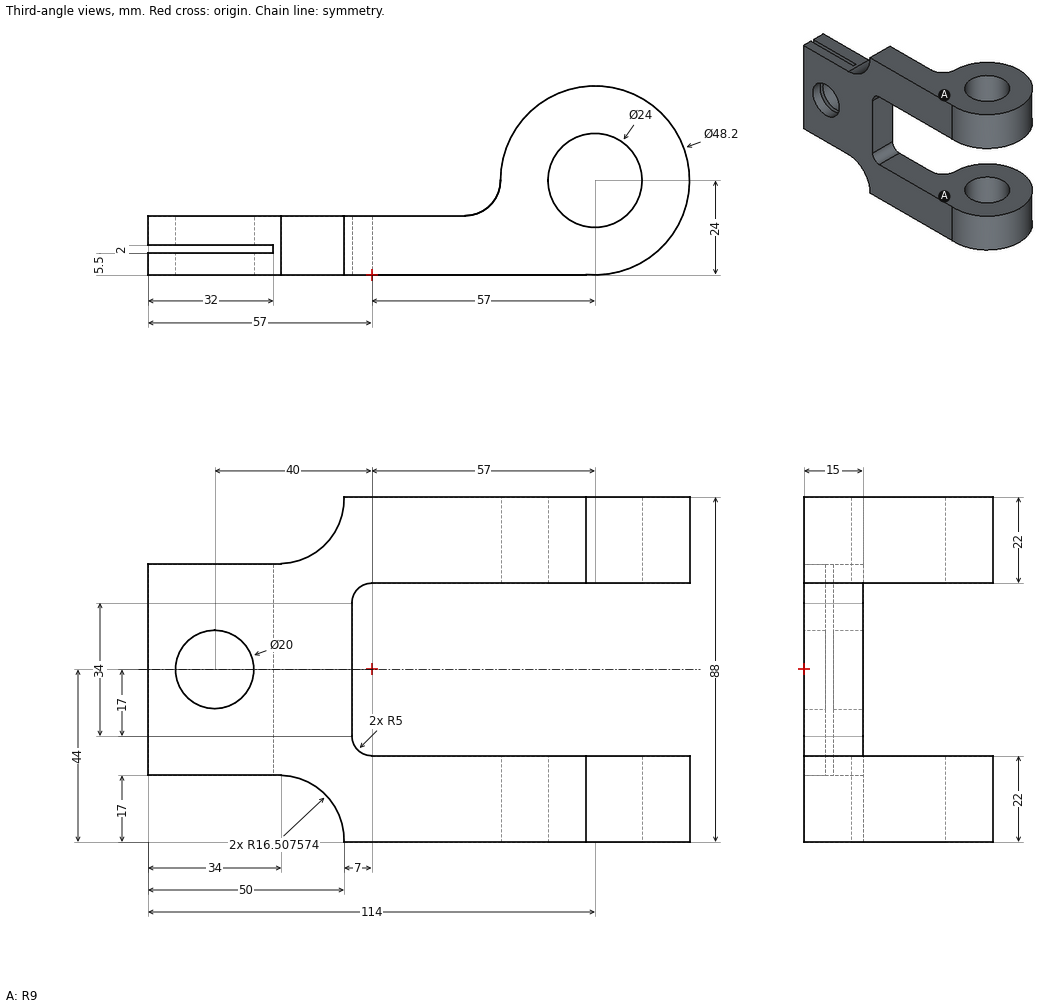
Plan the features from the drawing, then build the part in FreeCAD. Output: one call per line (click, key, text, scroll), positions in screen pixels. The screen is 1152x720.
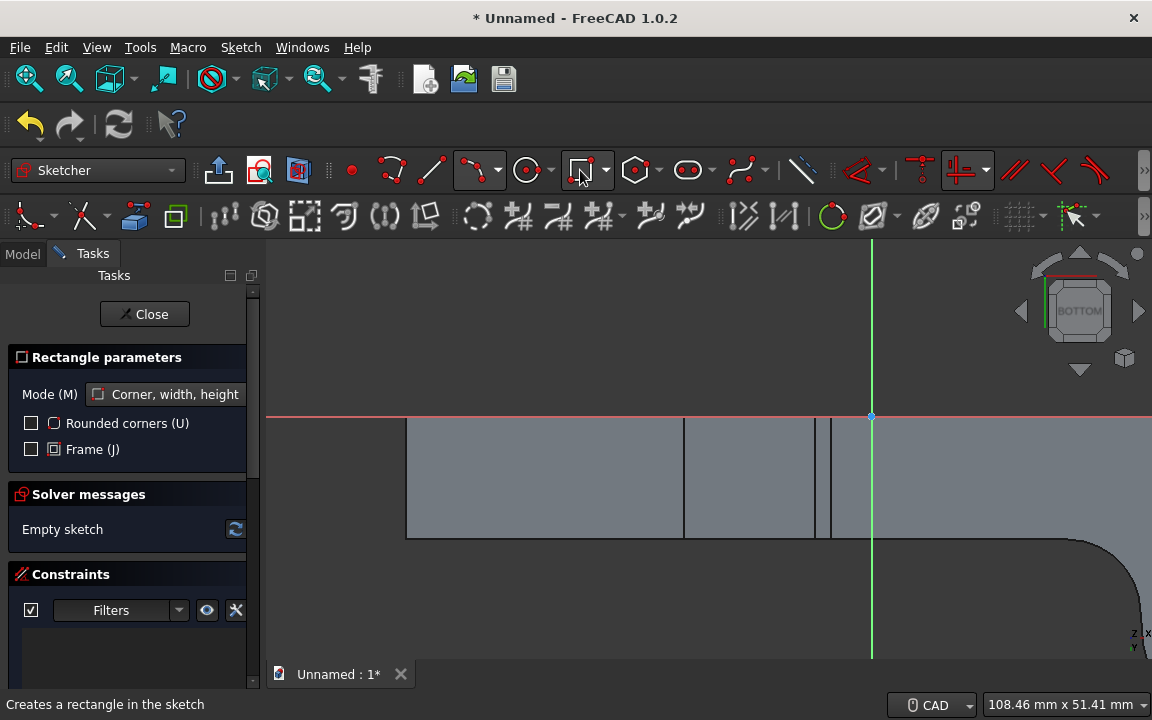
click(406, 462)
move(668, 478)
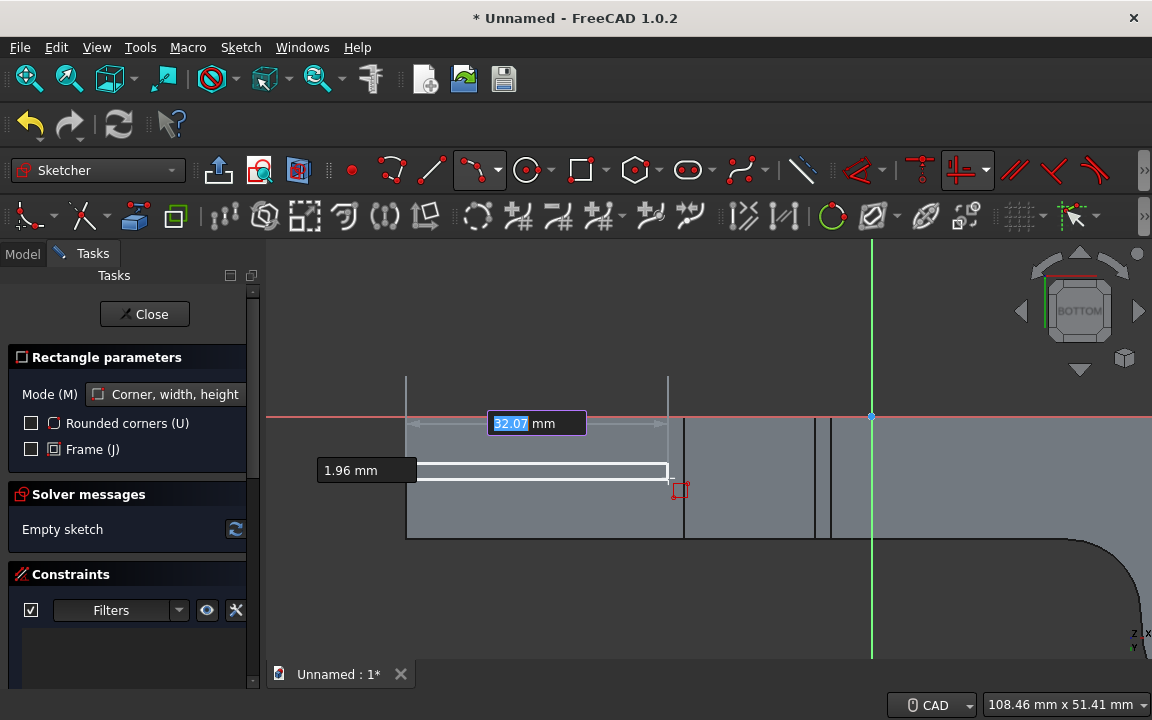
text(32)
key(Tab)
text(2)
key(Return)
key(Escape)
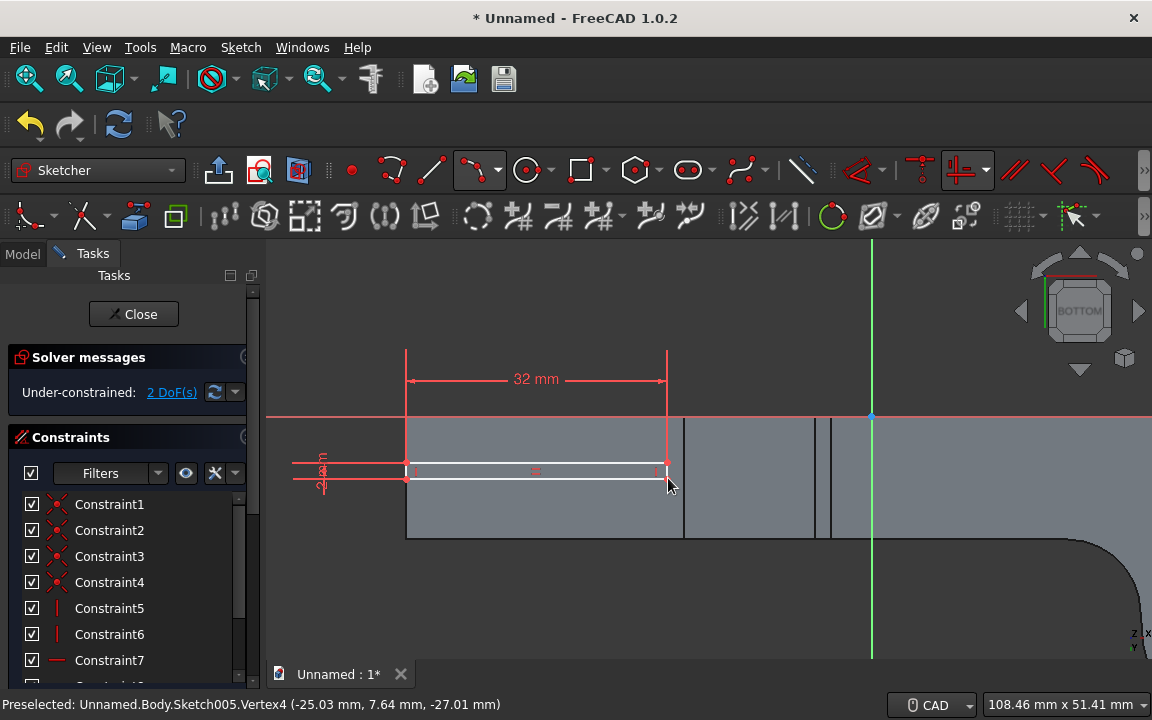
key(d)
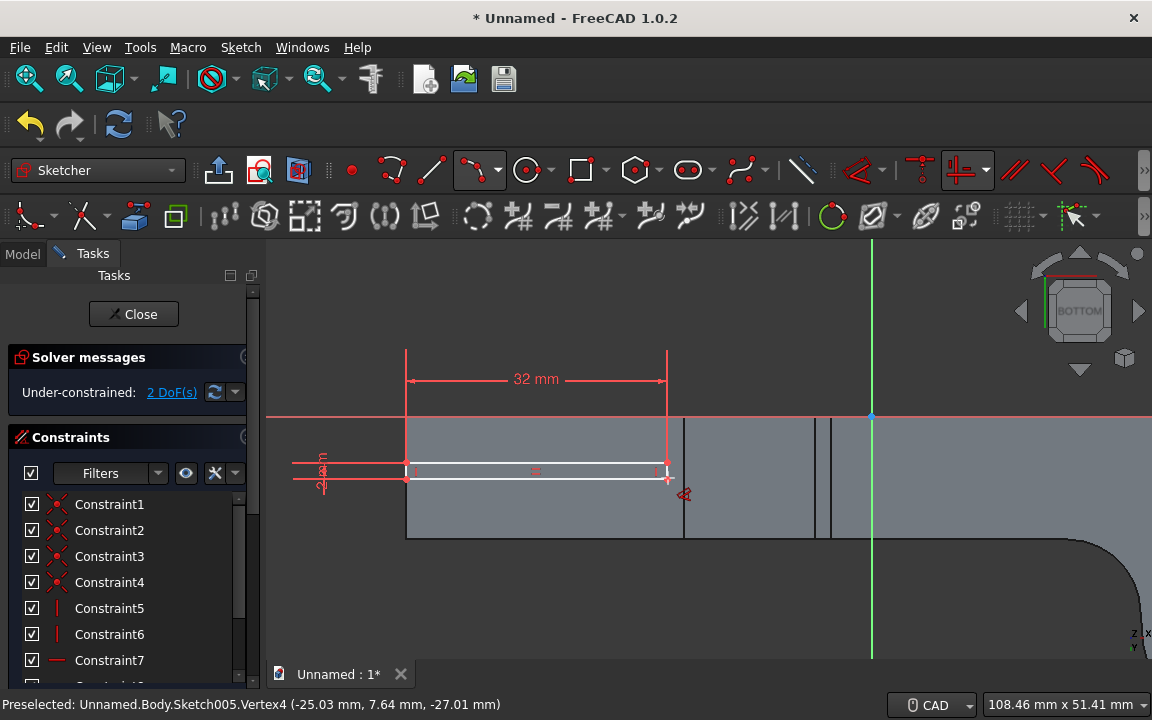
click(406, 463)
click(639, 383)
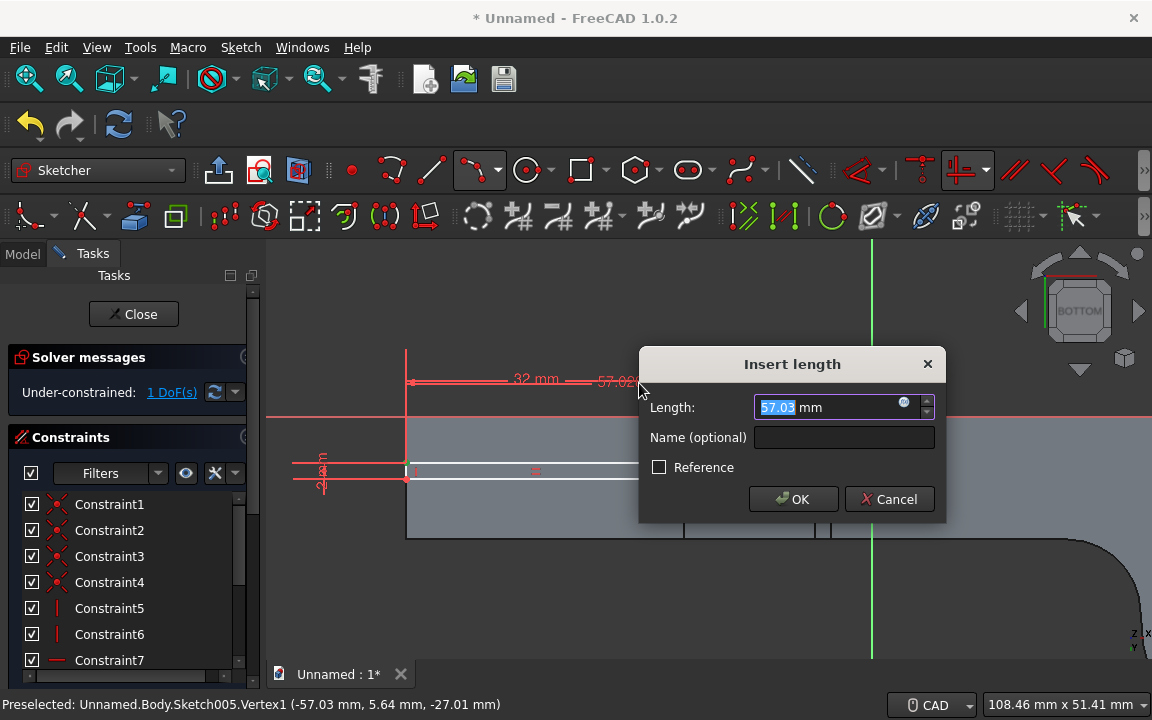
text(57)
key(Return)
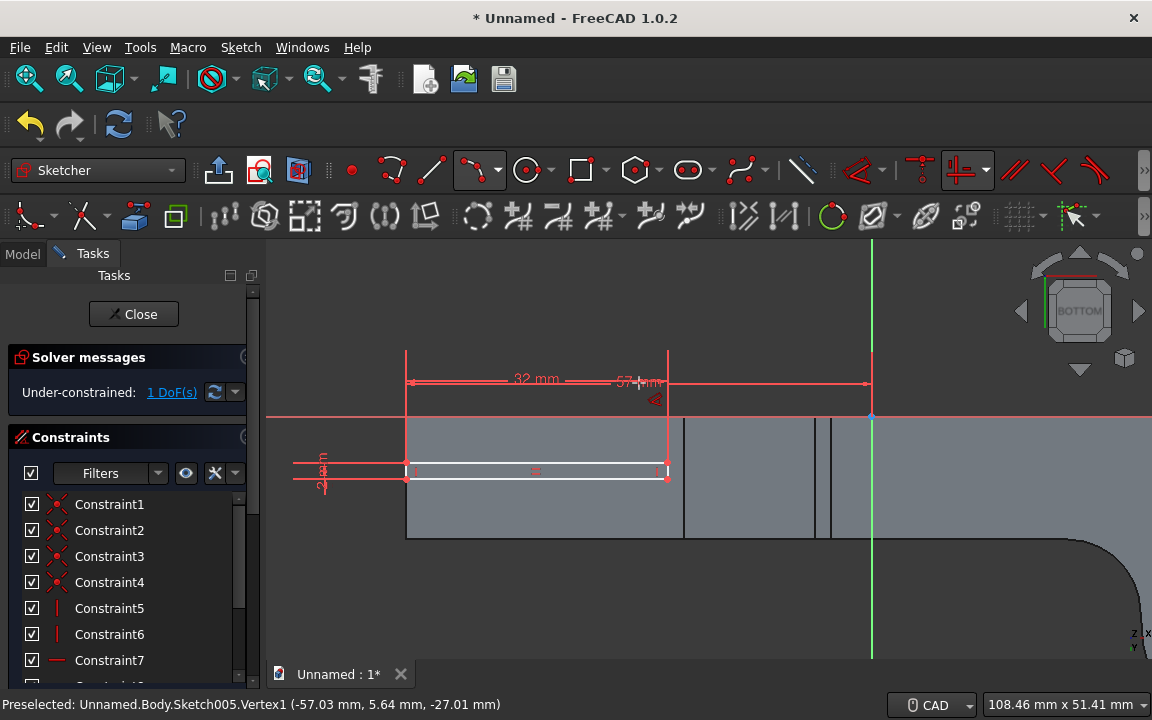
click(406, 463)
click(906, 440)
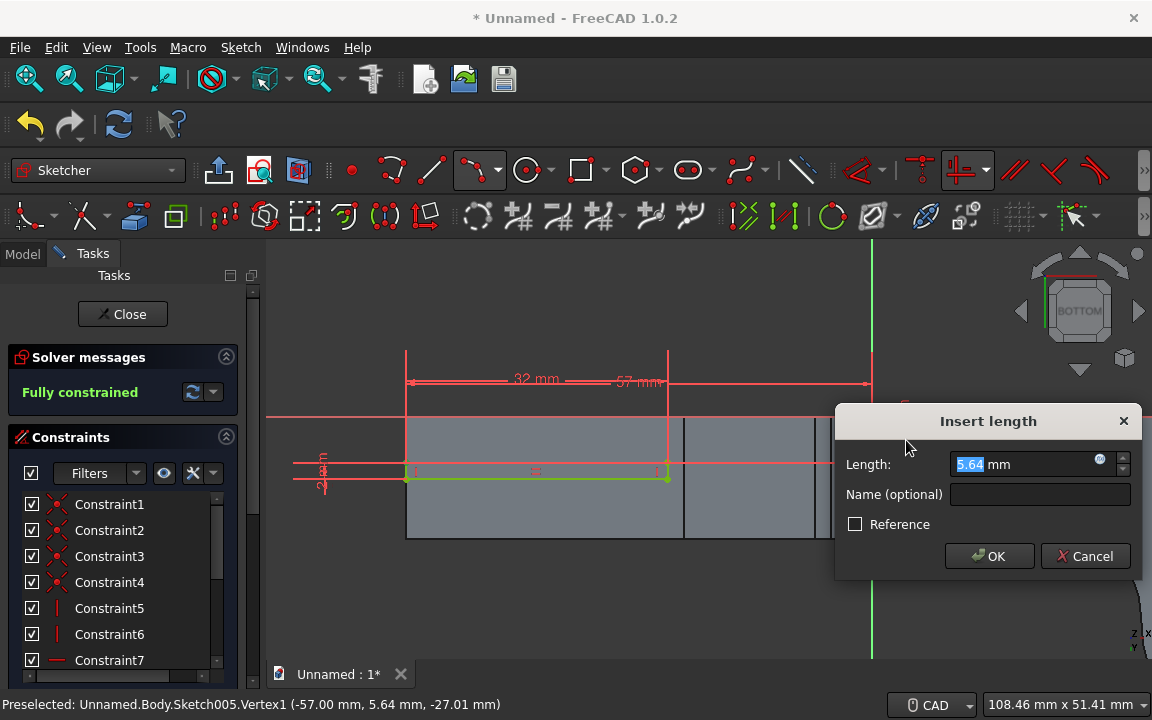
text(5.5)
key(Return)
key(Escape)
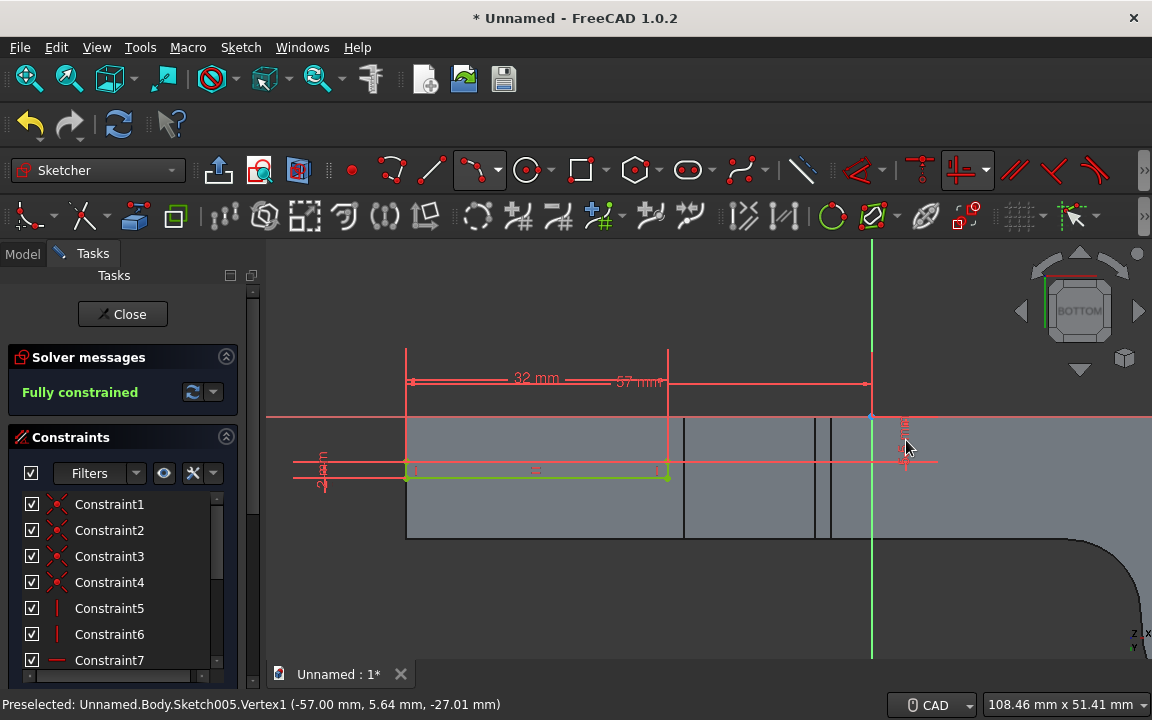
click(123, 314)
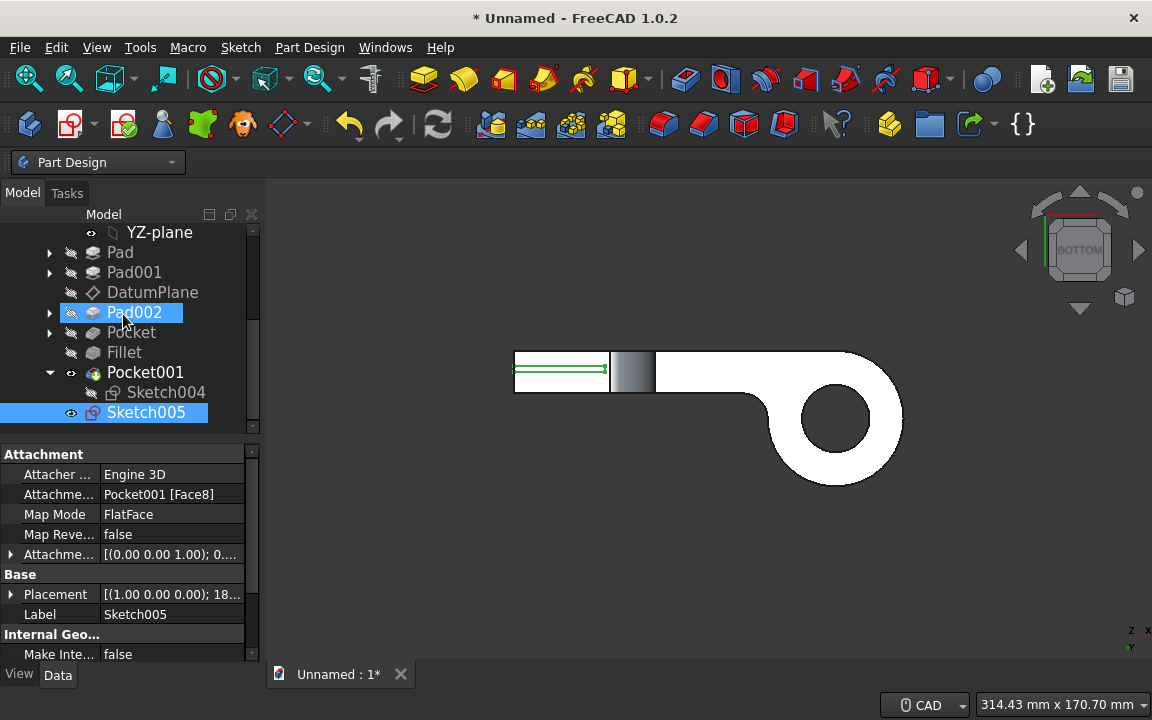
click(686, 80)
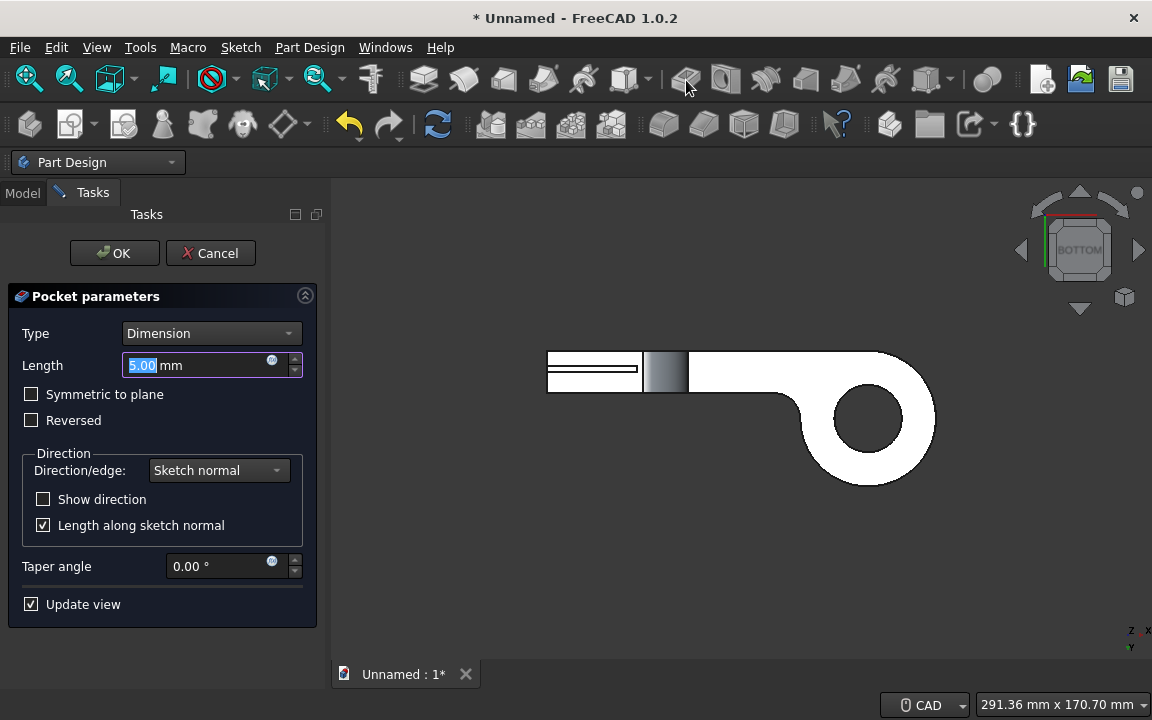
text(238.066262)
key(Tab)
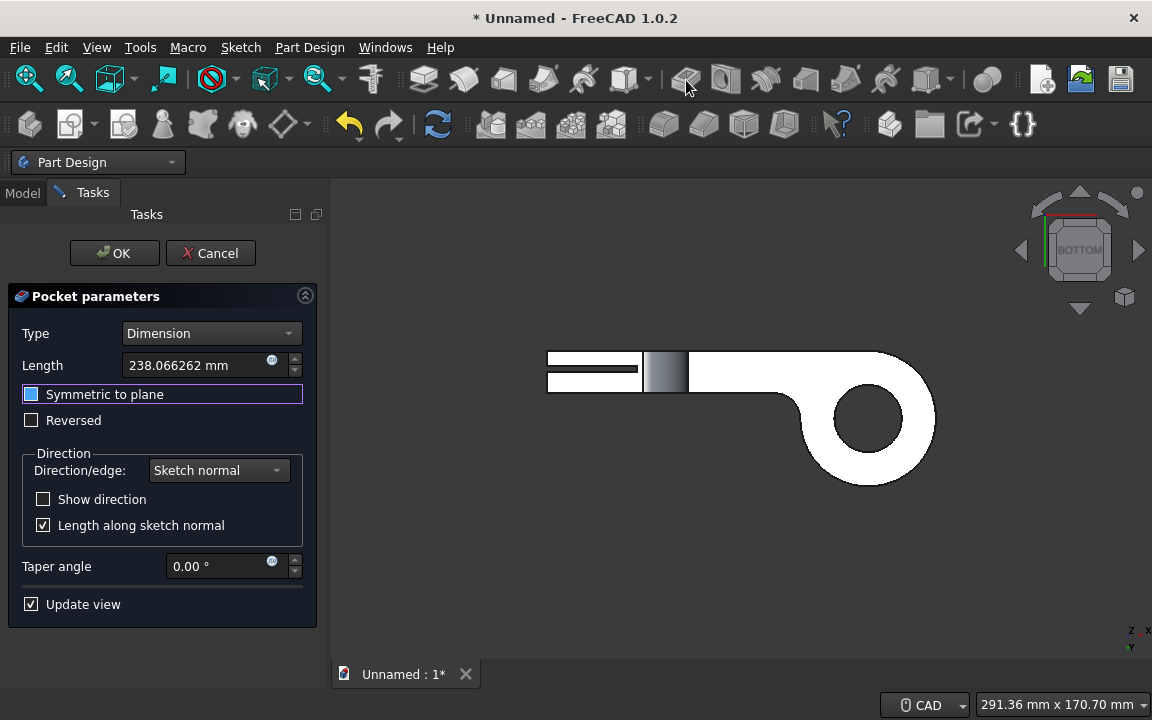
click(30, 394)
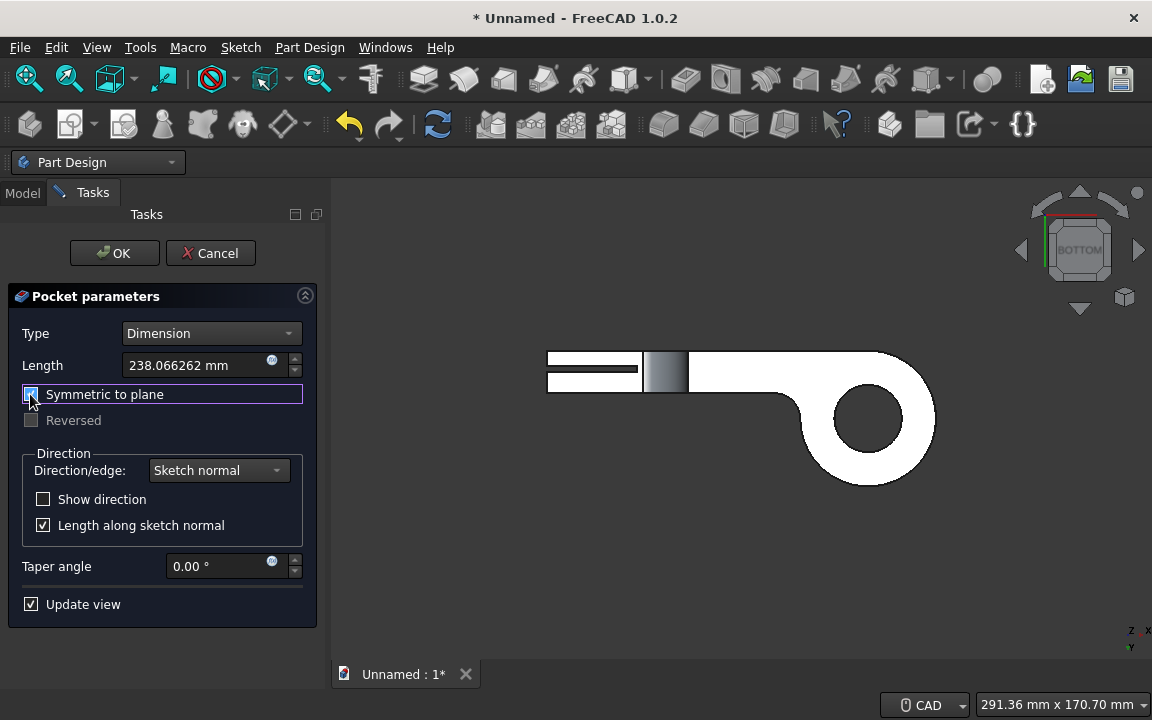
click(115, 253)